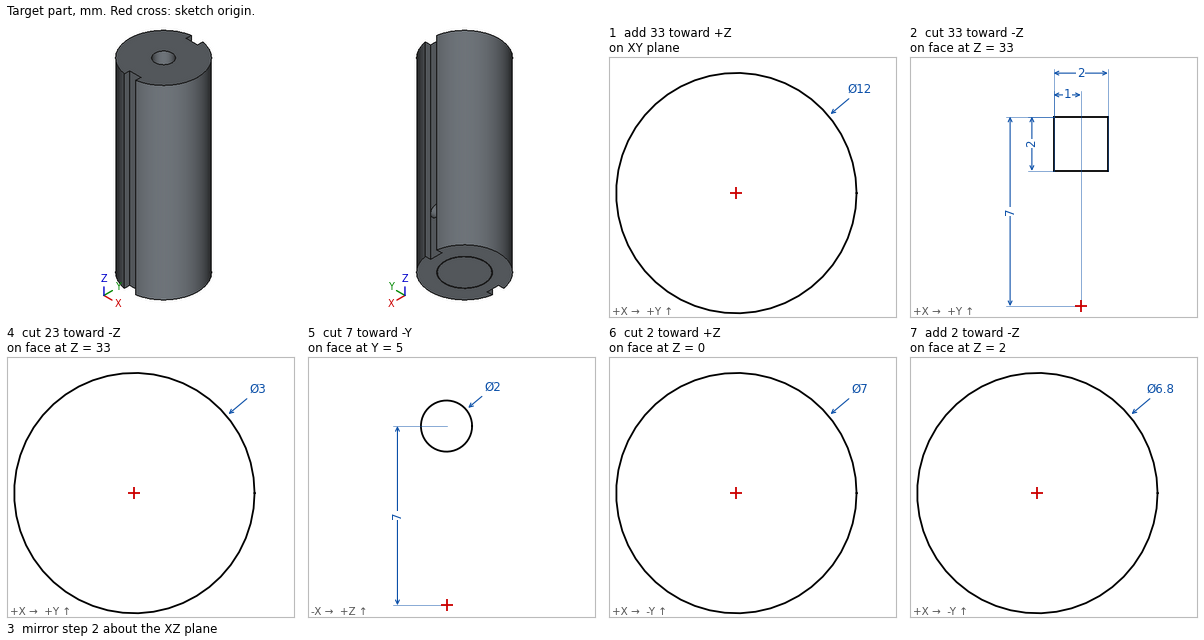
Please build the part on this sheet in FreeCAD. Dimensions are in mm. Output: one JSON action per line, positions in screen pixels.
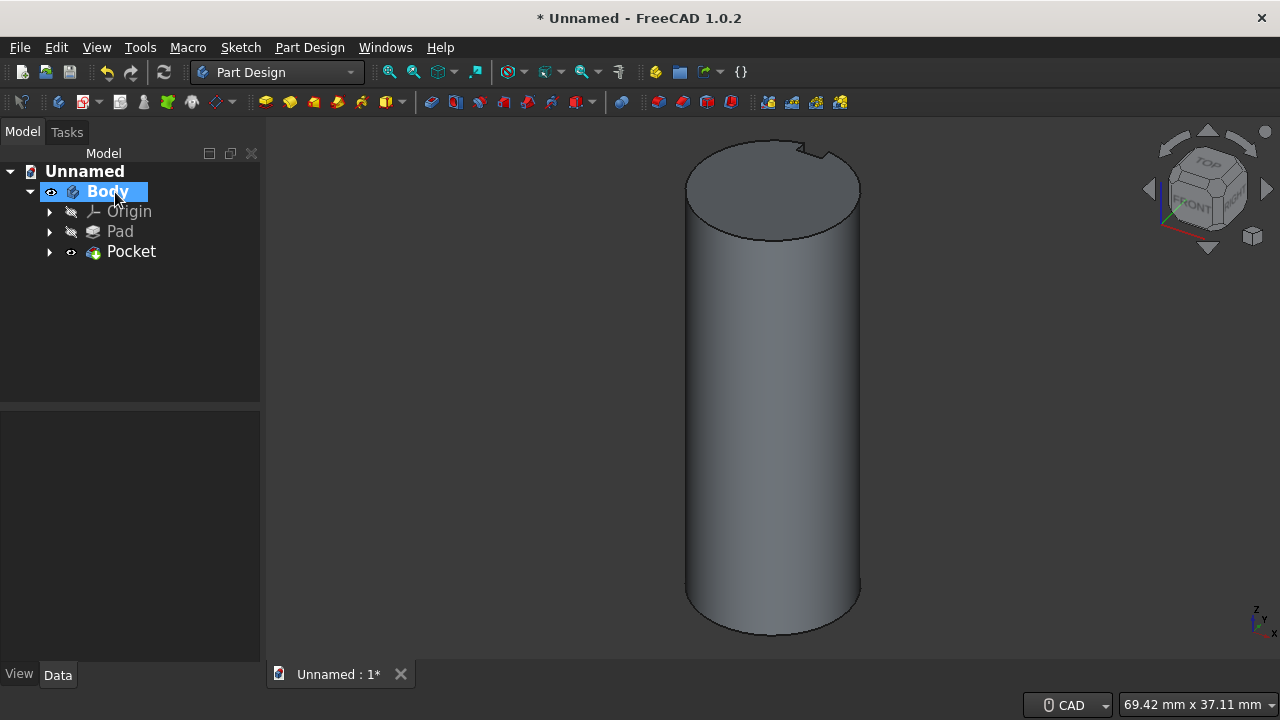
{"action": "left_click", "coordinate": [116, 252]}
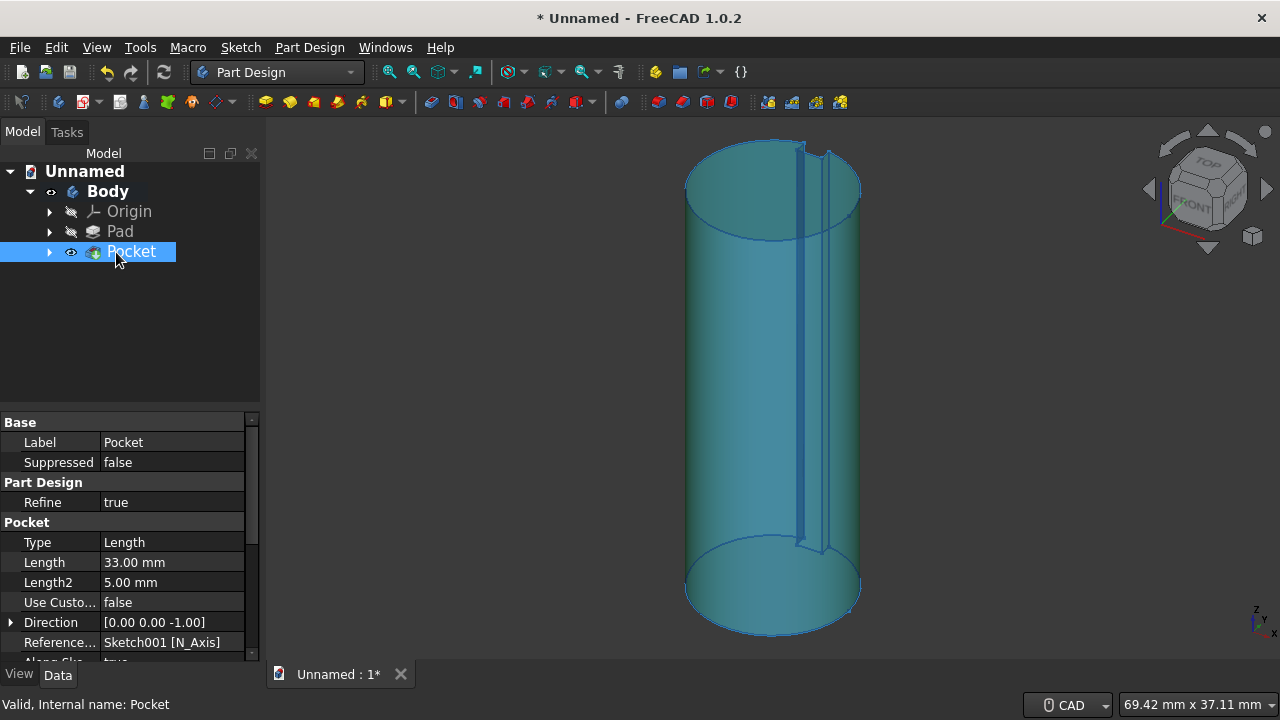
{"action": "left_click", "coordinate": [768, 102]}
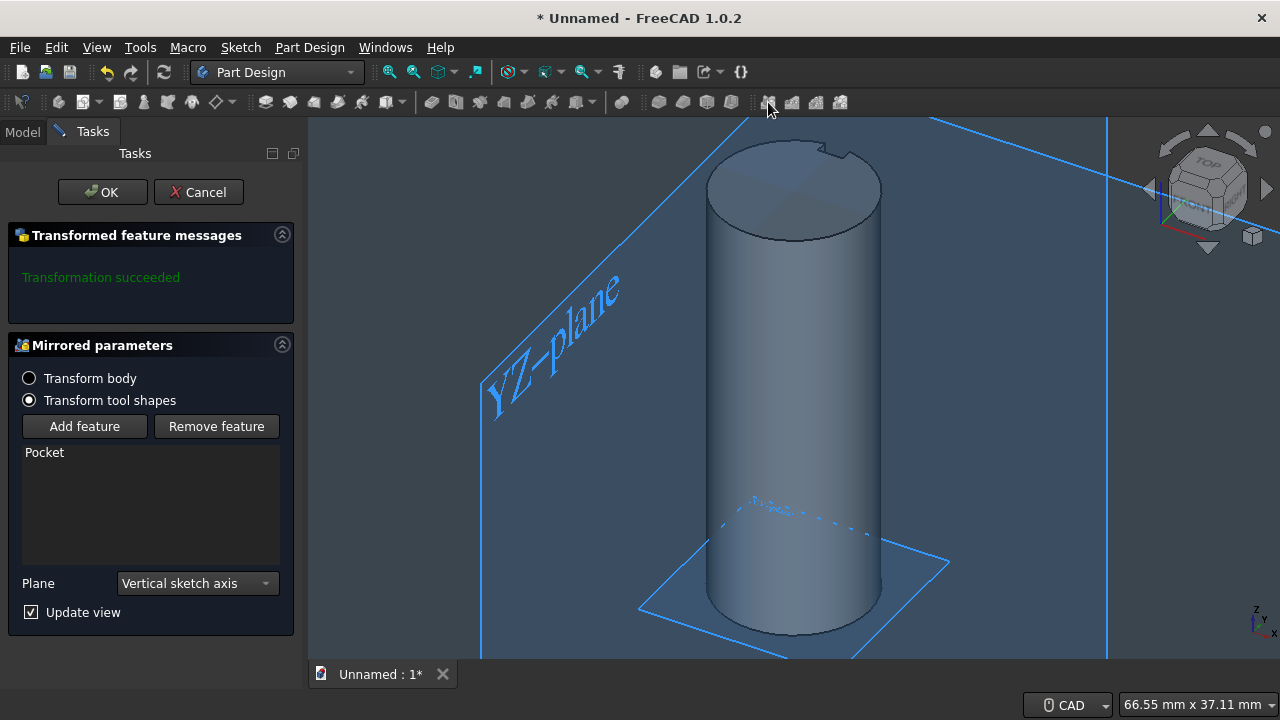
{"action": "left_click", "coordinate": [198, 584]}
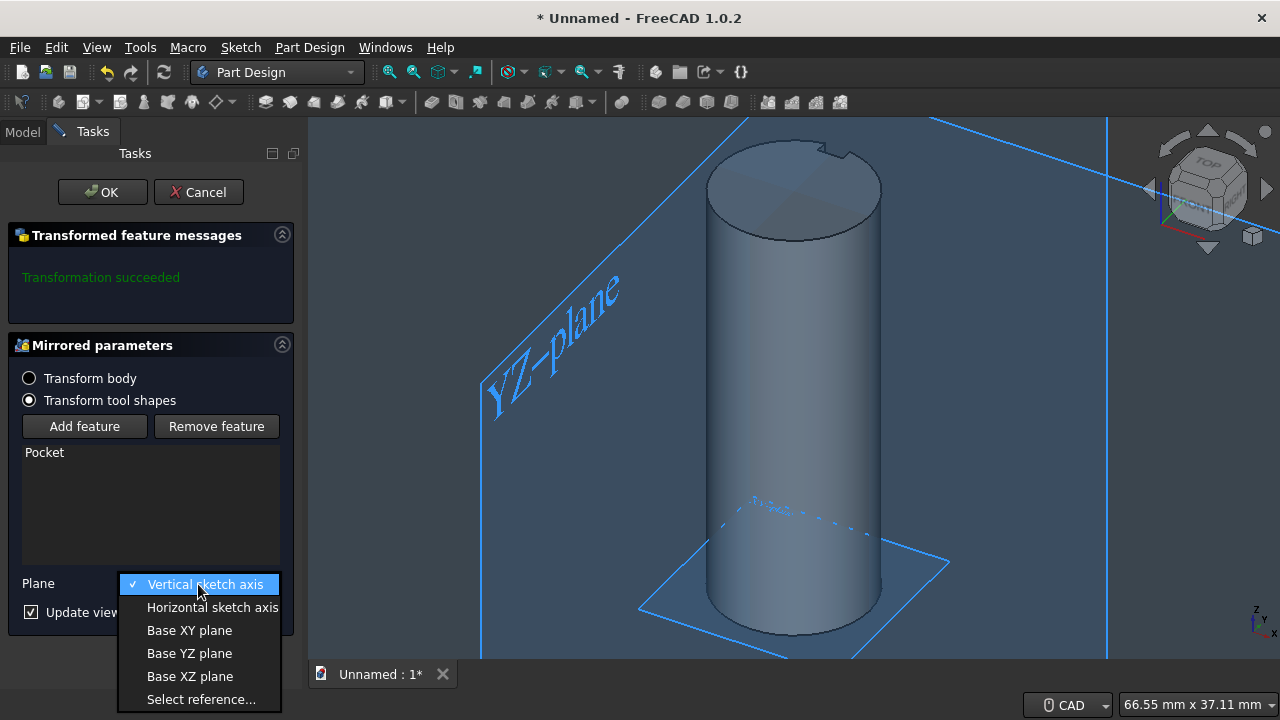
{"action": "left_click", "coordinate": [198, 676]}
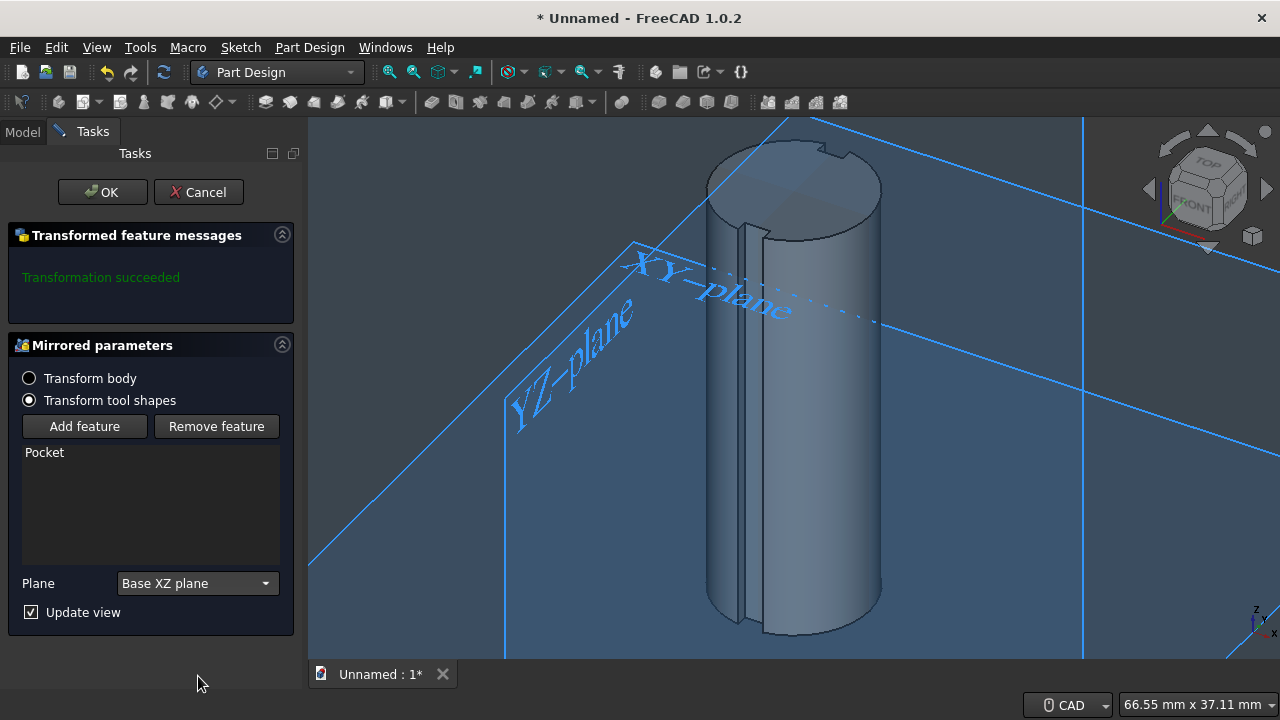
{"action": "left_click", "coordinate": [103, 192]}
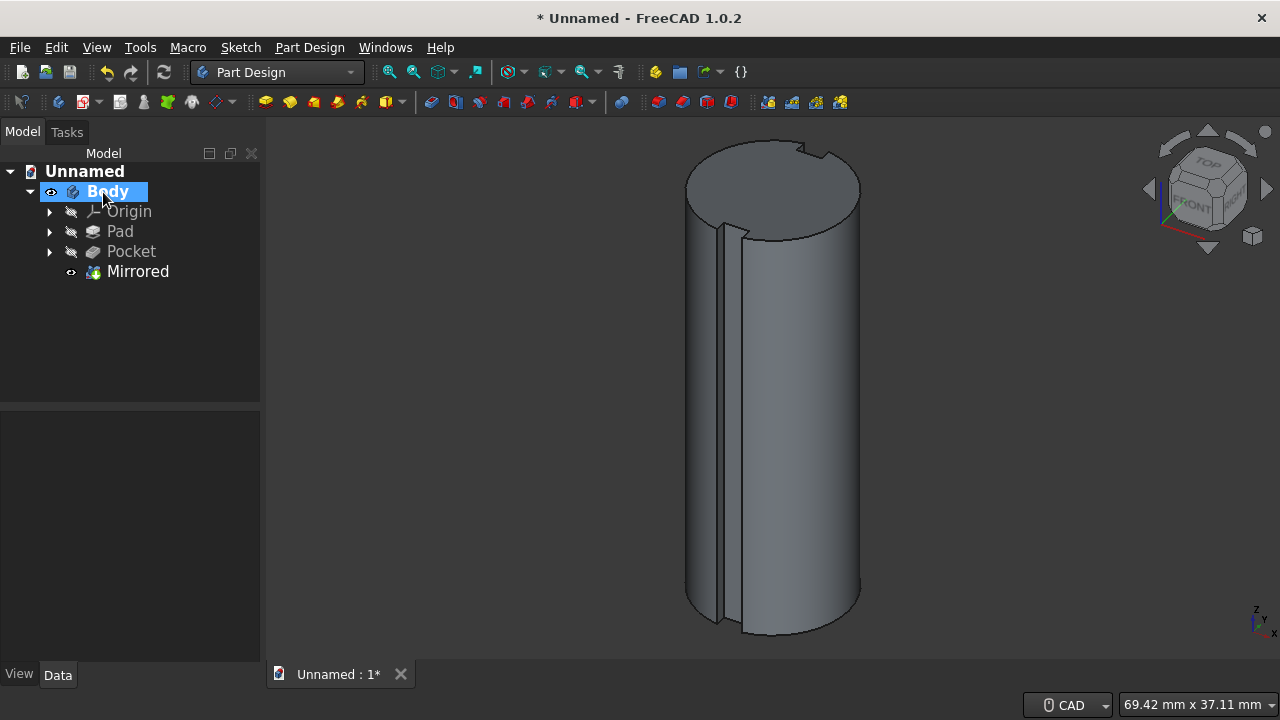
{"action": "left_click", "coordinate": [773, 190]}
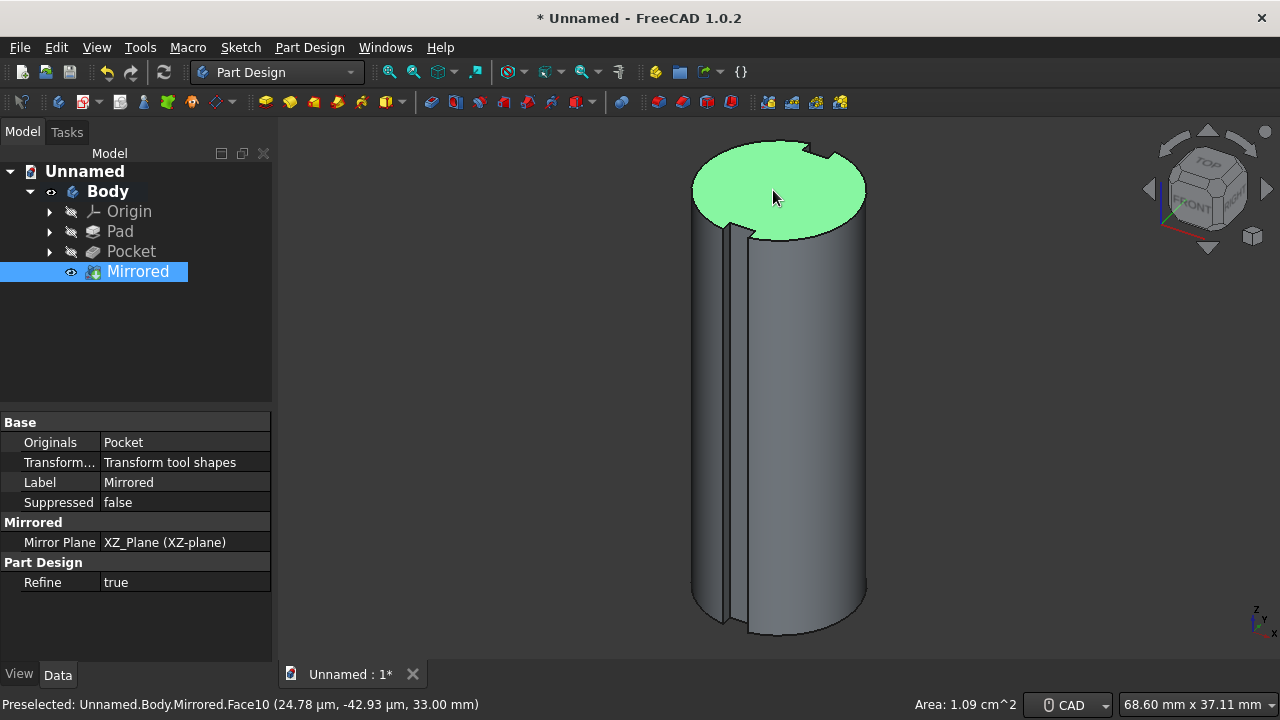
{"action": "left_click", "coordinate": [84, 102]}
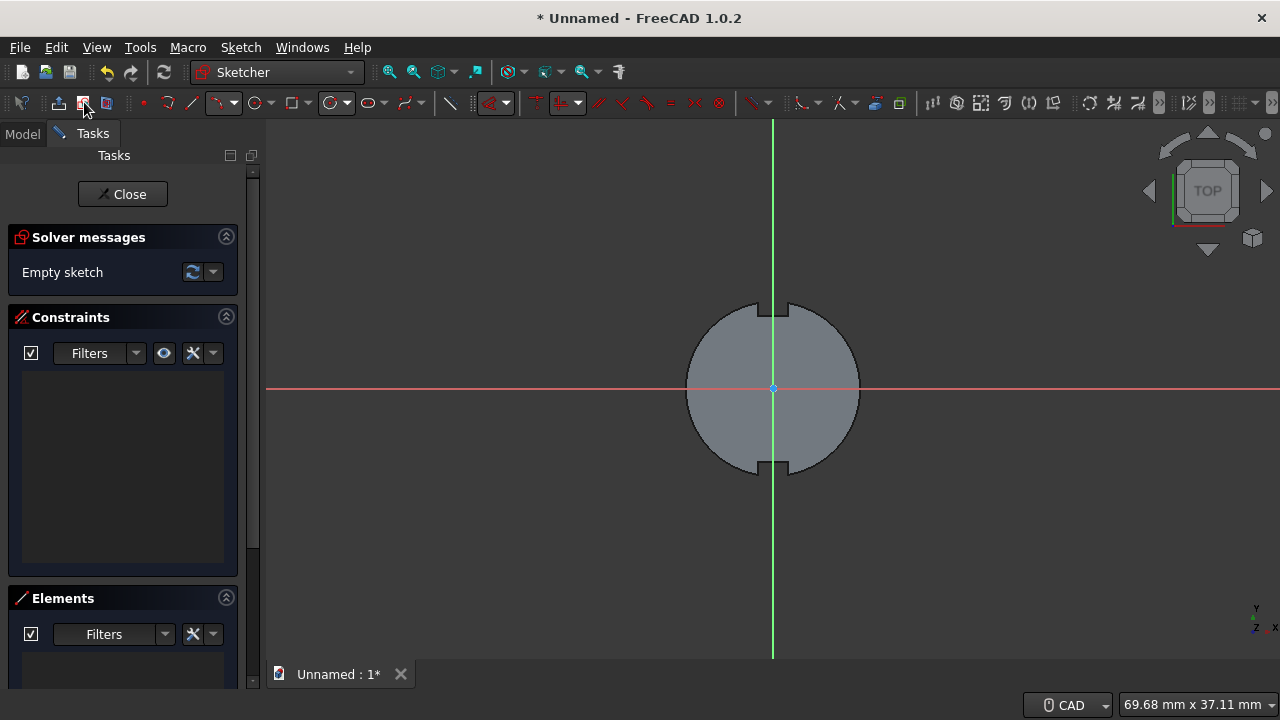
{"action": "scroll", "coordinate": [784, 389], "scroll_direction": "up", "scroll_amount": 10}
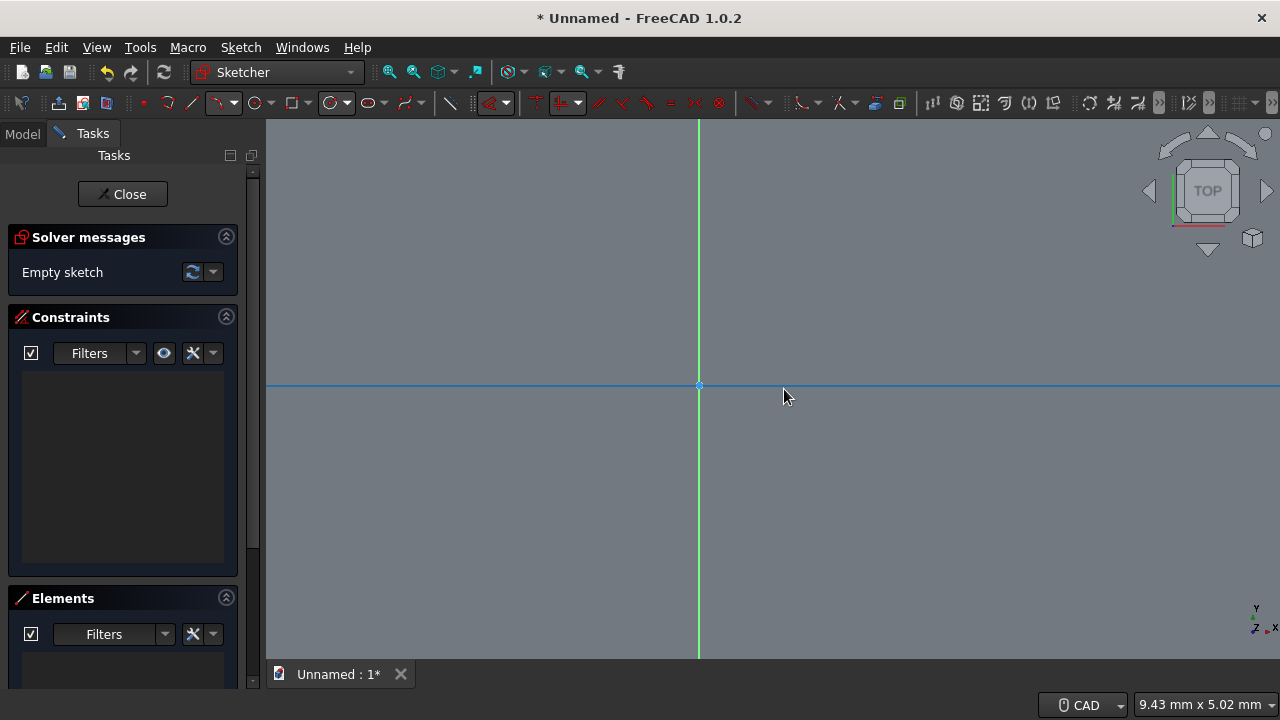
{"action": "left_click", "coordinate": [256, 104]}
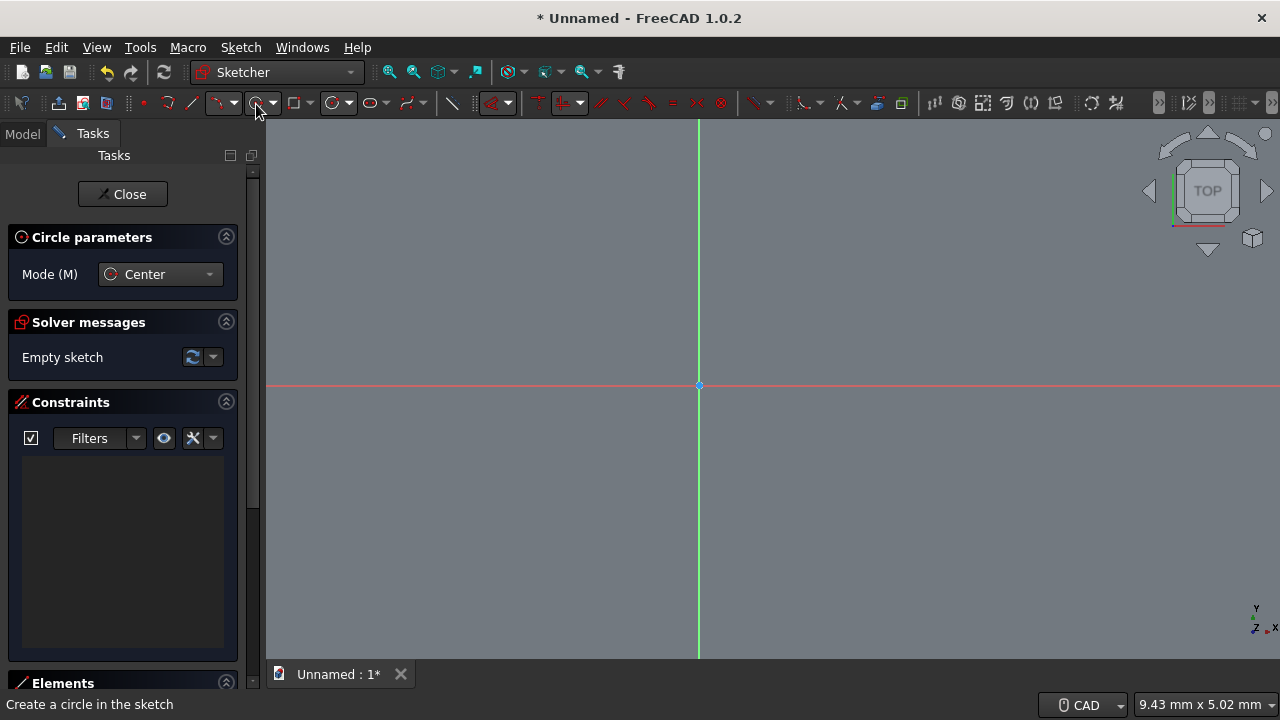
{"action": "left_click", "coordinate": [699, 386]}
{"action": "left_click", "coordinate": [814, 272]}
{"action": "key", "text": "Escape"}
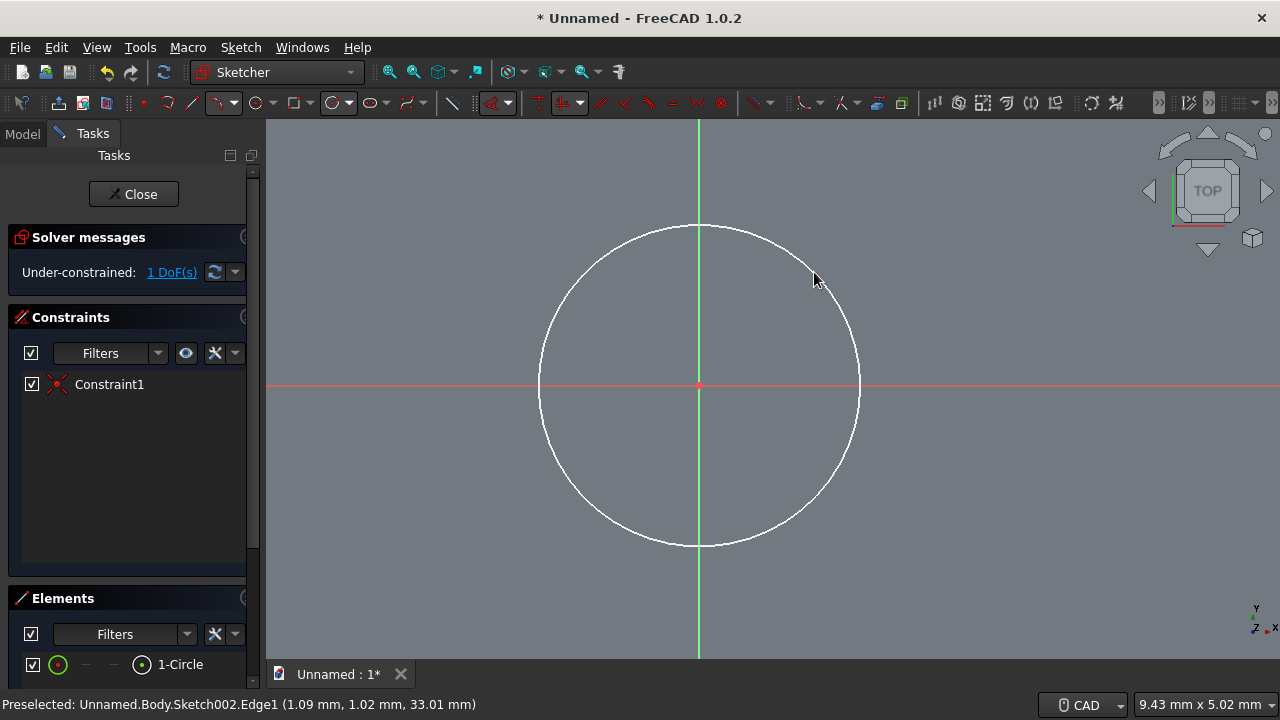
{"action": "key", "text": "d"}